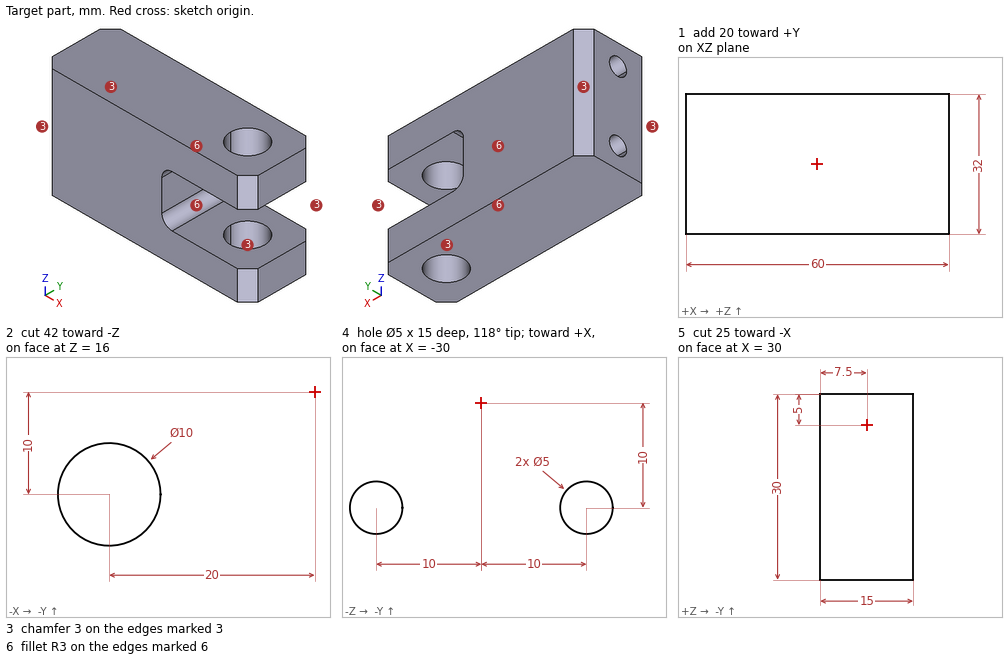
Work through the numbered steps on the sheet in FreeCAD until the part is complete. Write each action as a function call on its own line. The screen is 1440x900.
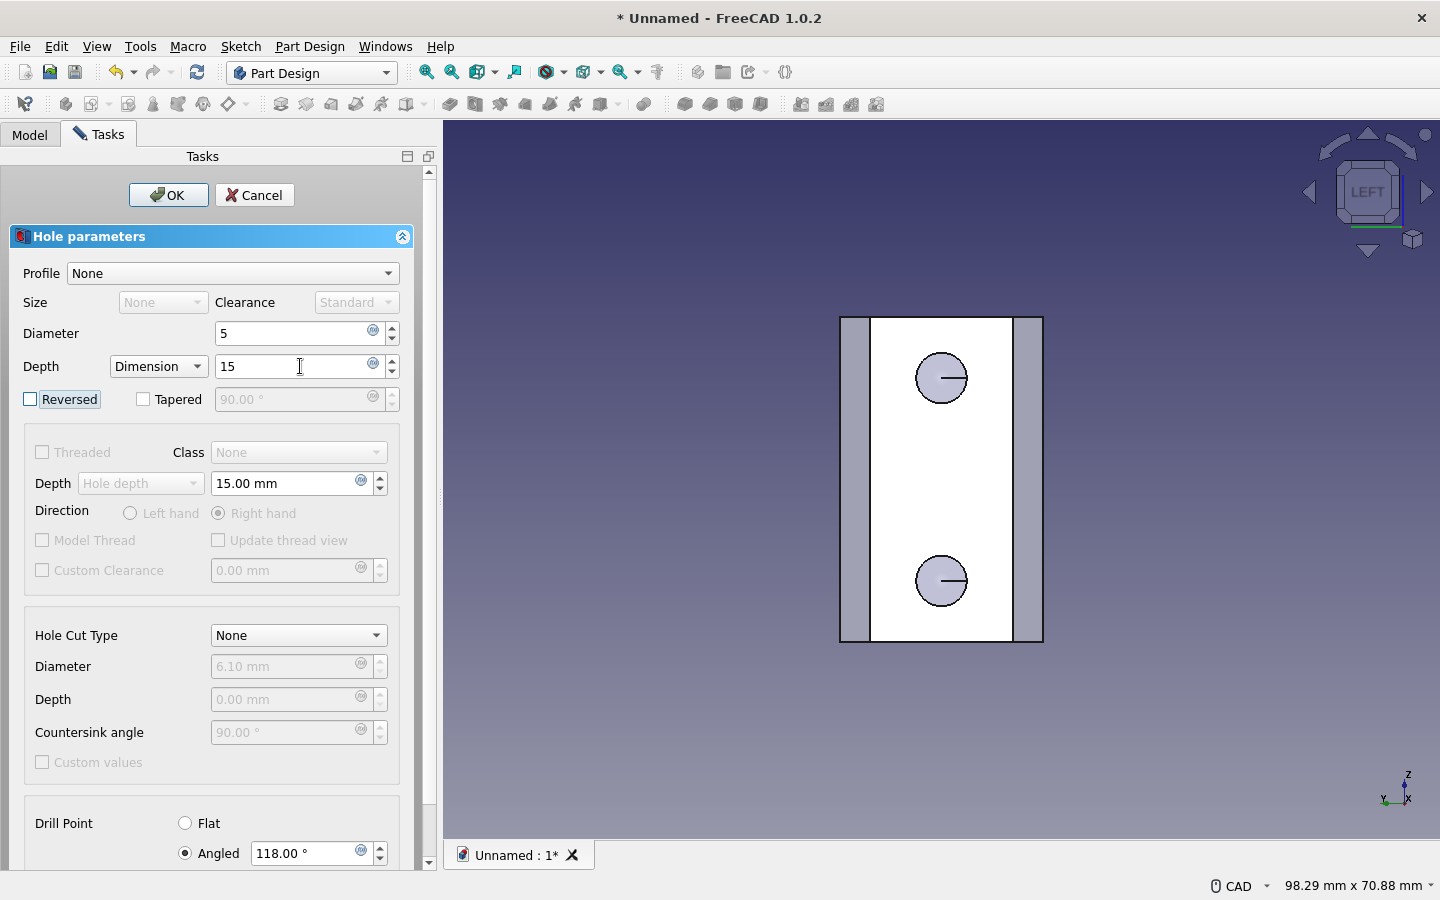
click(169, 195)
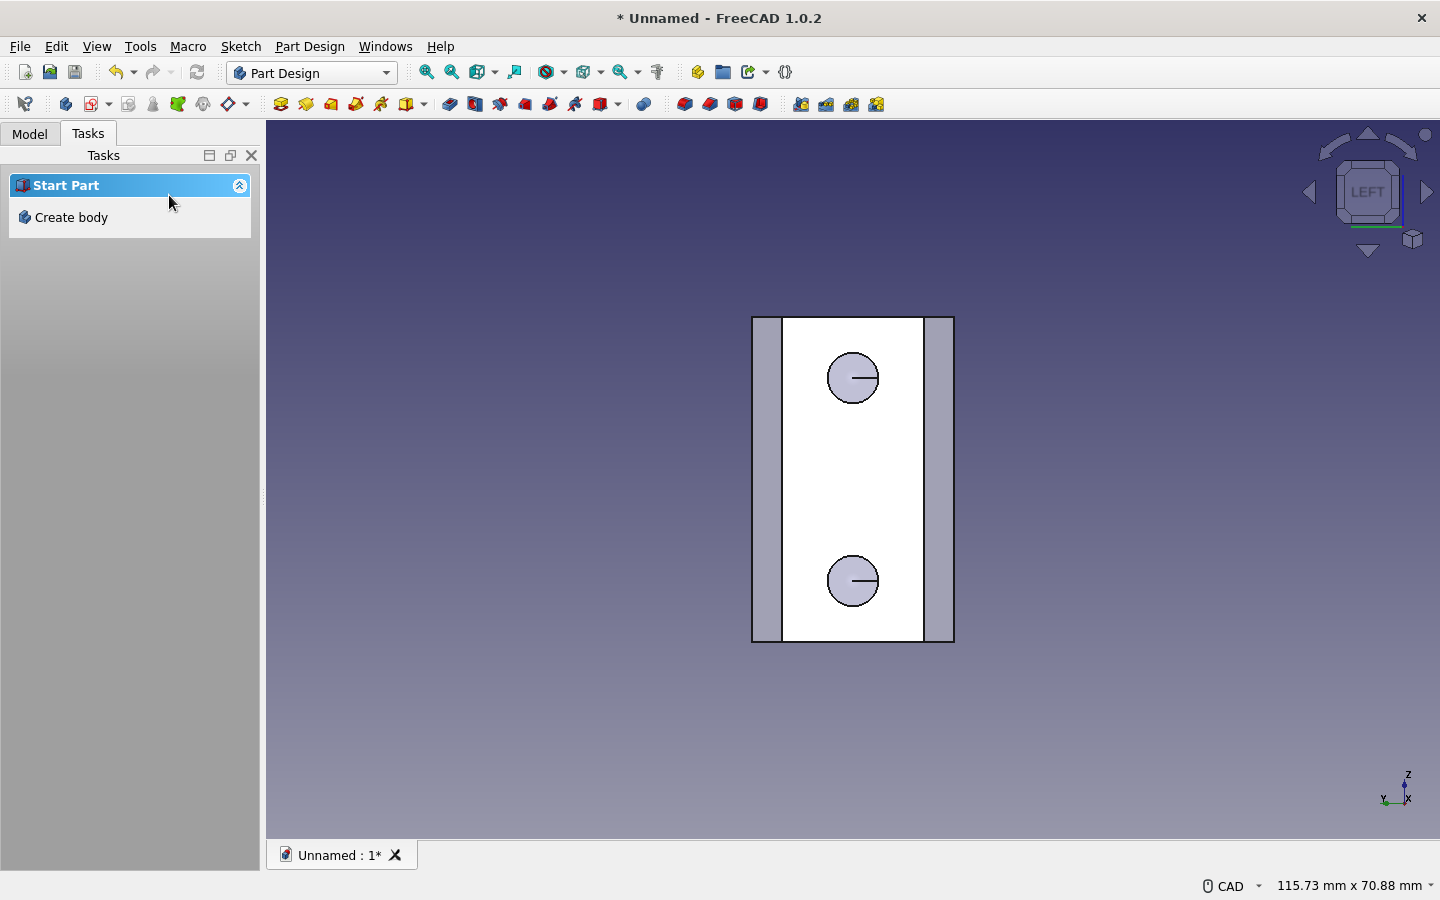
key(0)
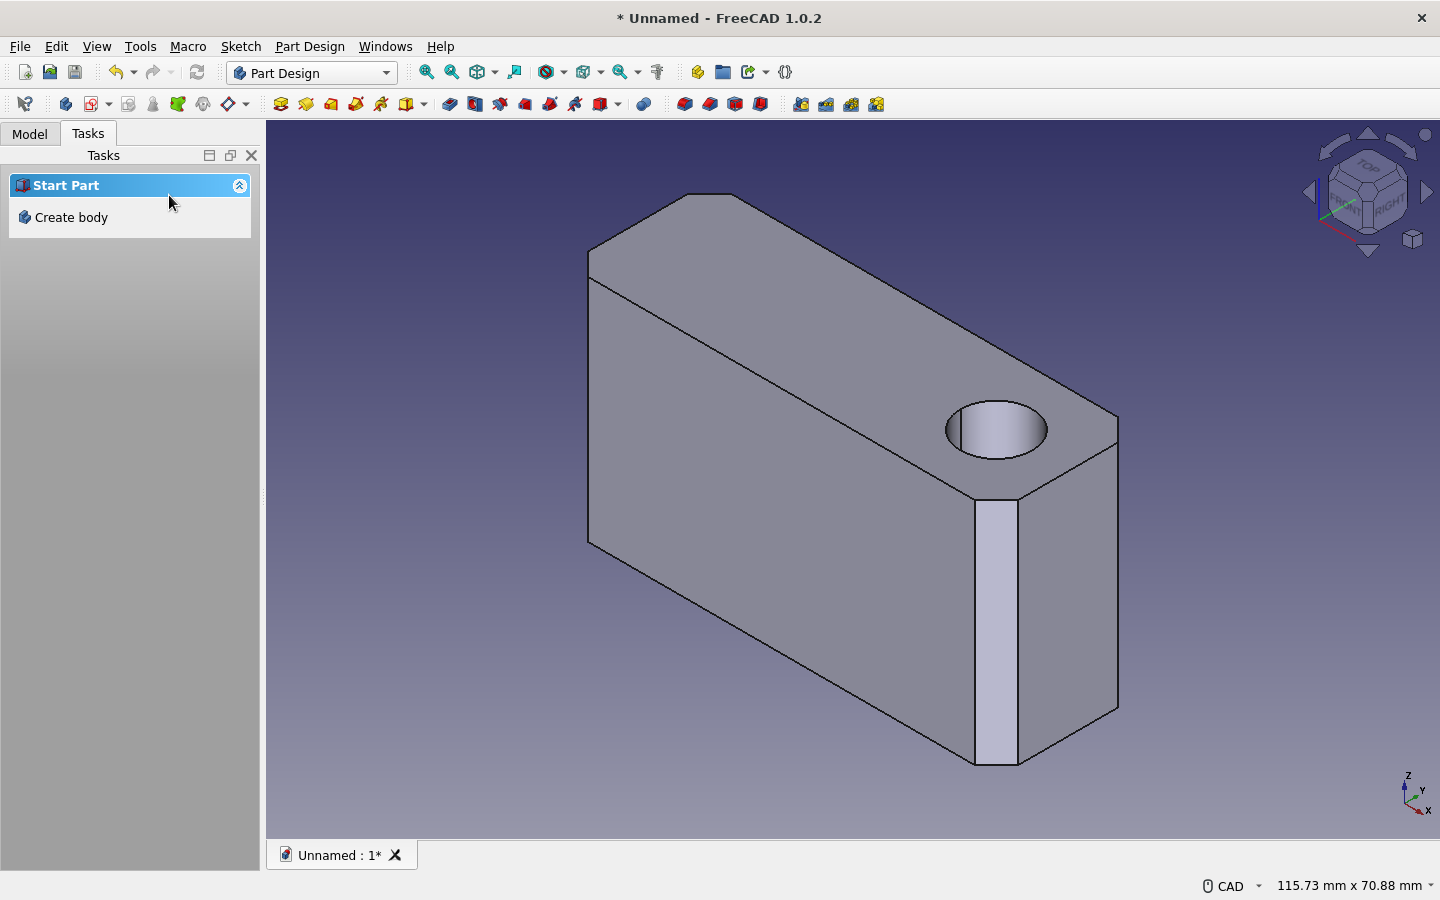
click(1068, 565)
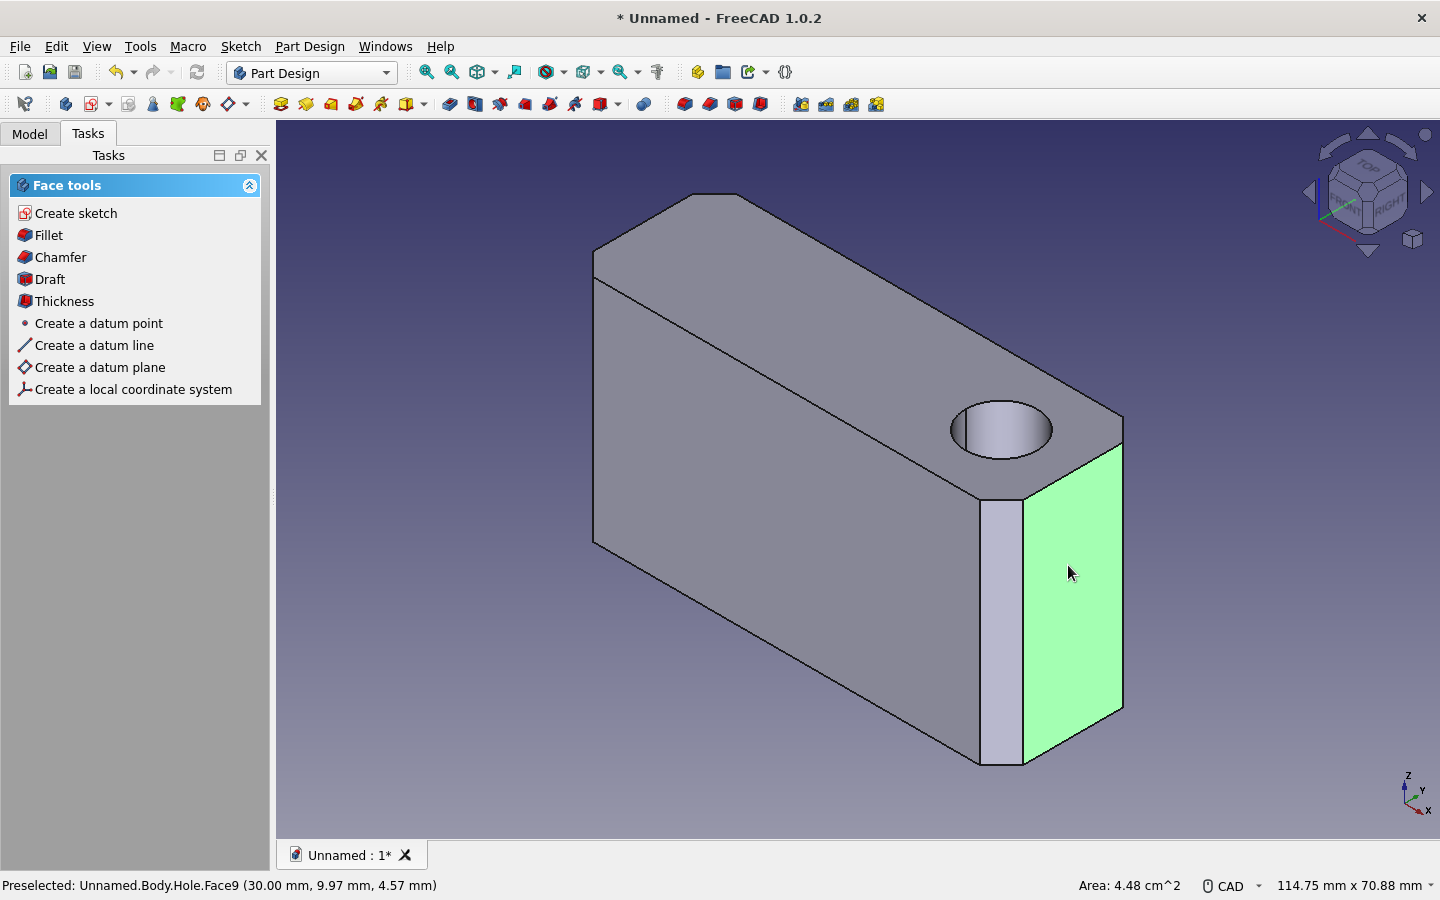
click(90, 104)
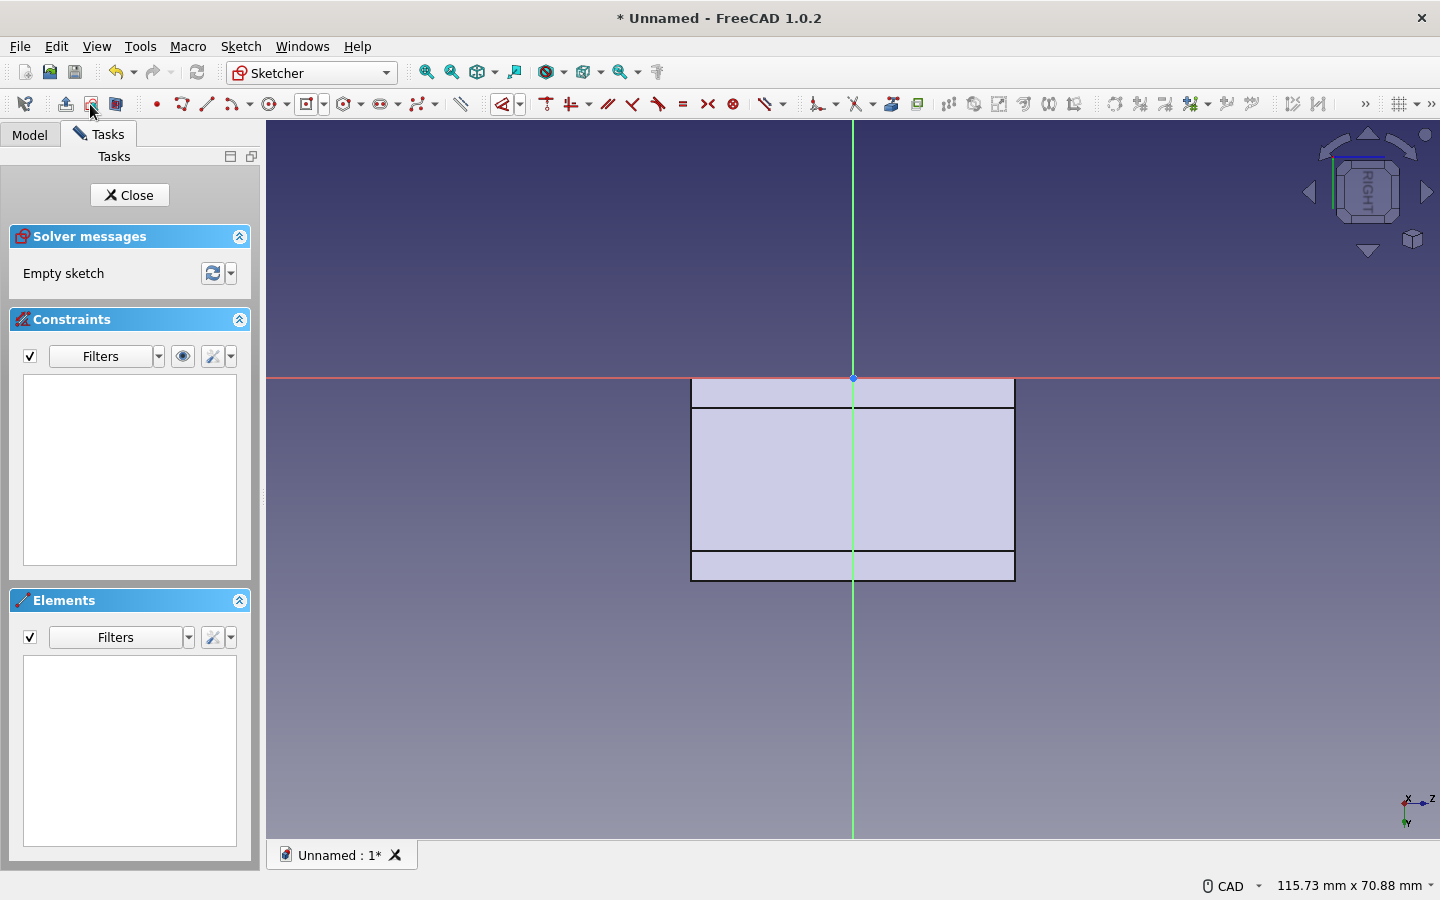
scroll(992, 479, up, 2)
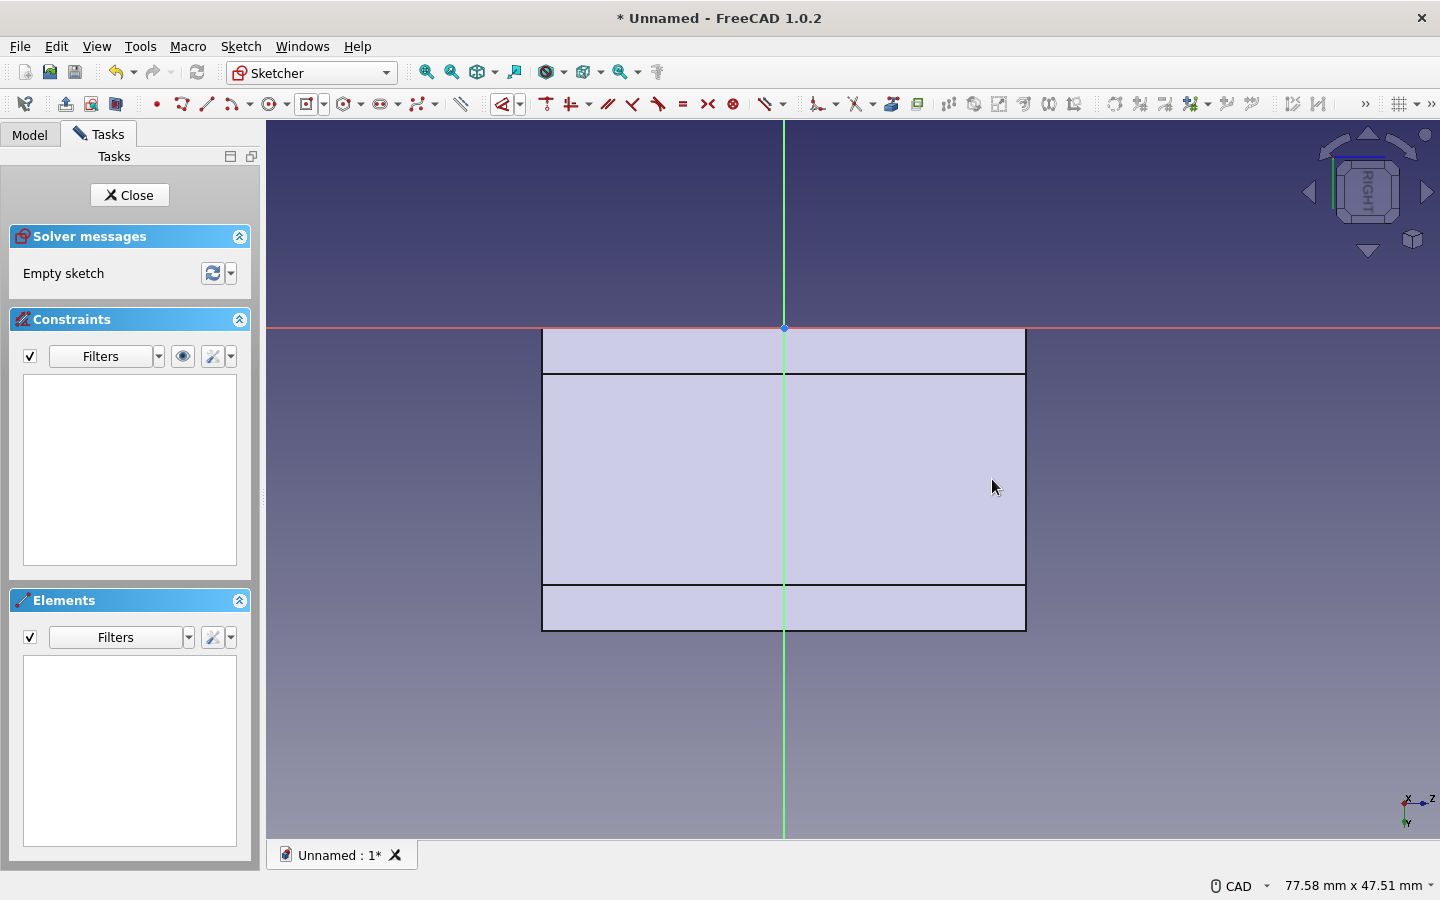
key(g)
key(r)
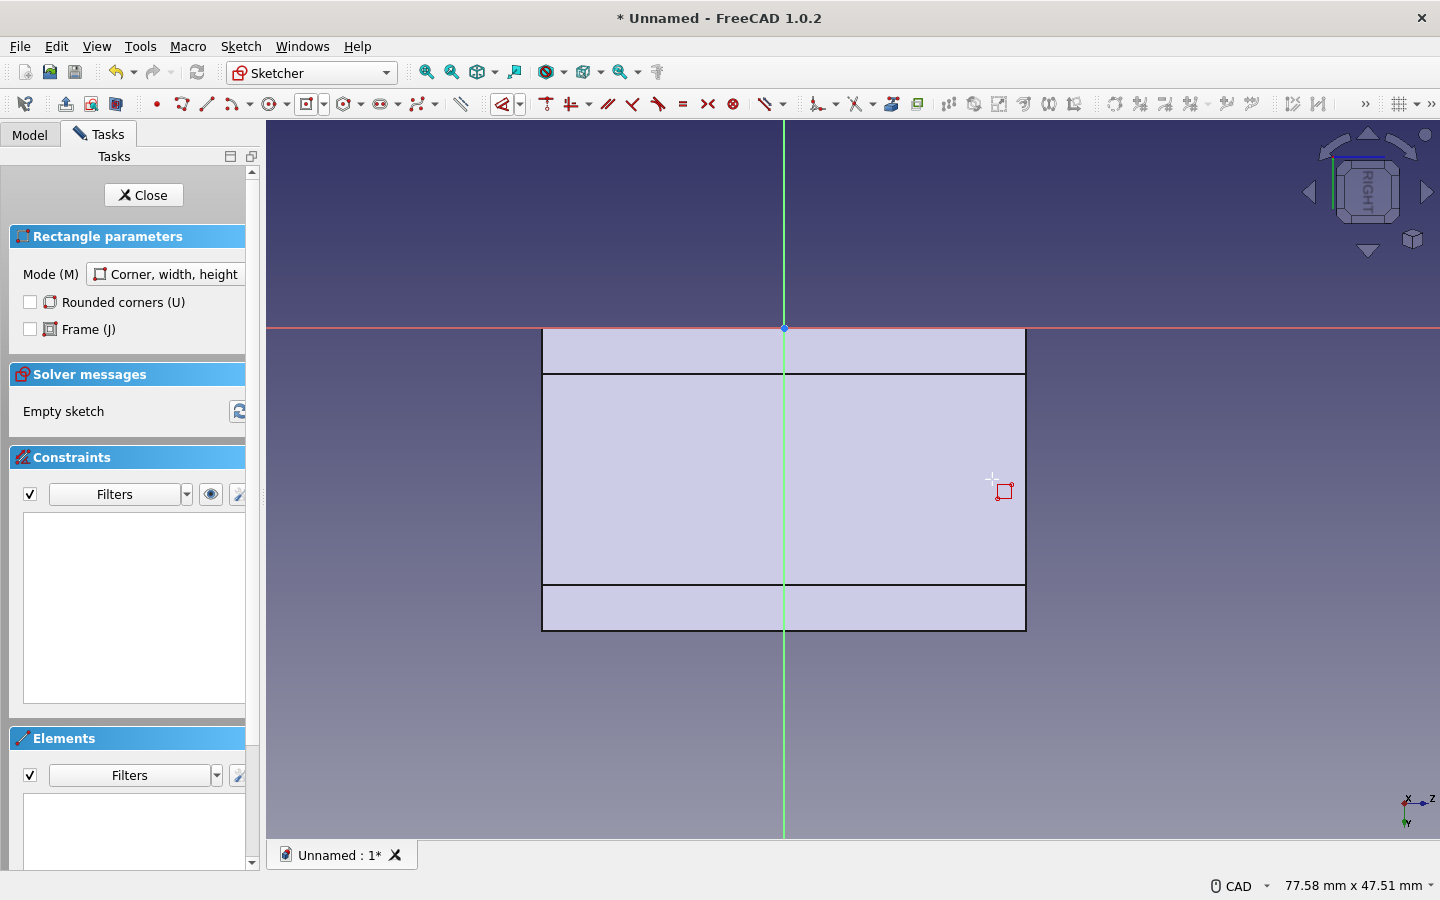
click(671, 253)
click(898, 706)
key(Escape)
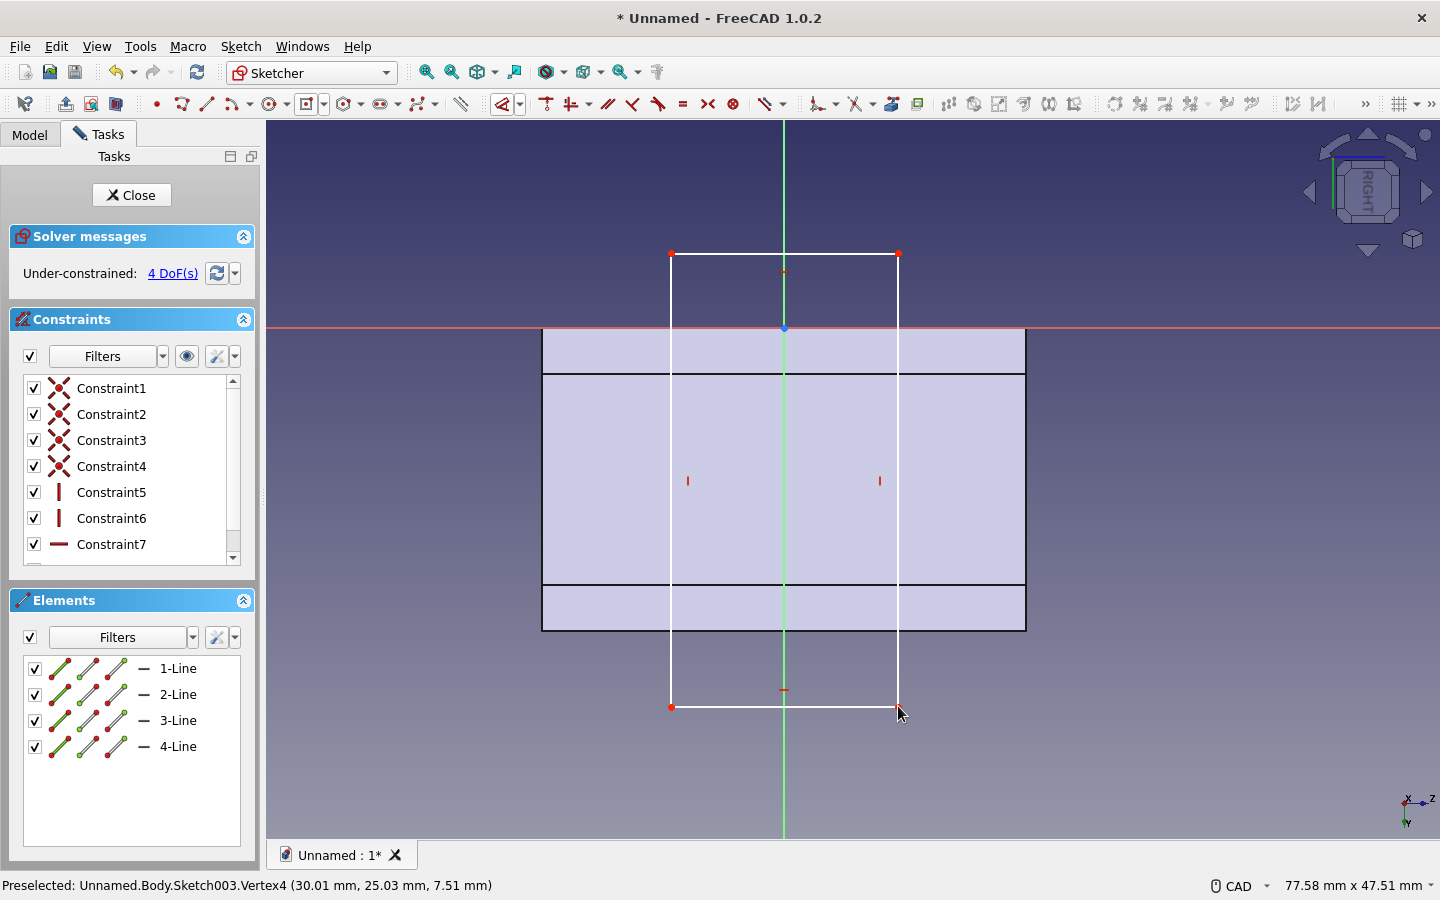
click(671, 390)